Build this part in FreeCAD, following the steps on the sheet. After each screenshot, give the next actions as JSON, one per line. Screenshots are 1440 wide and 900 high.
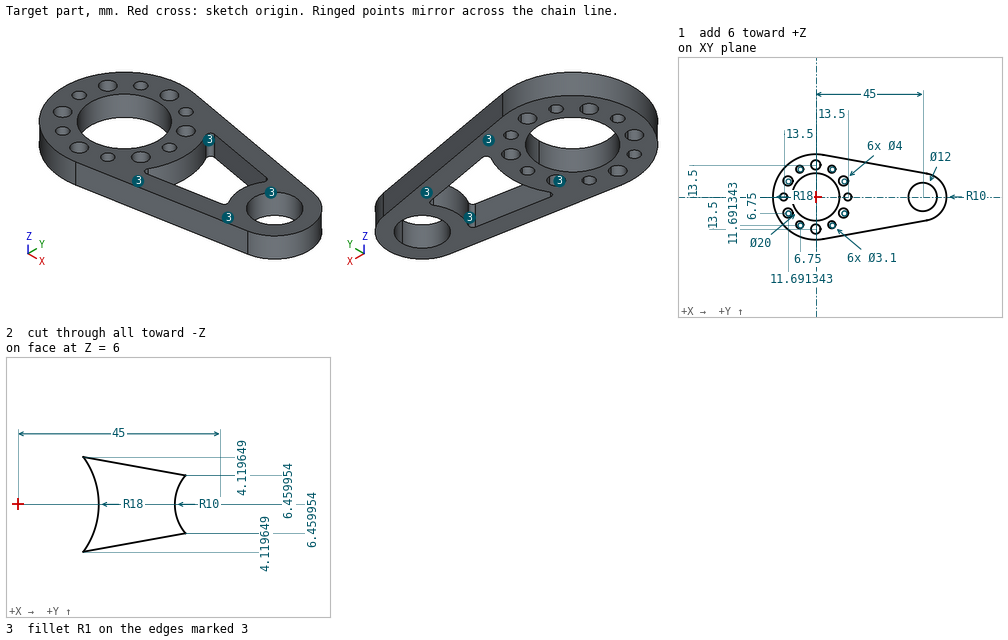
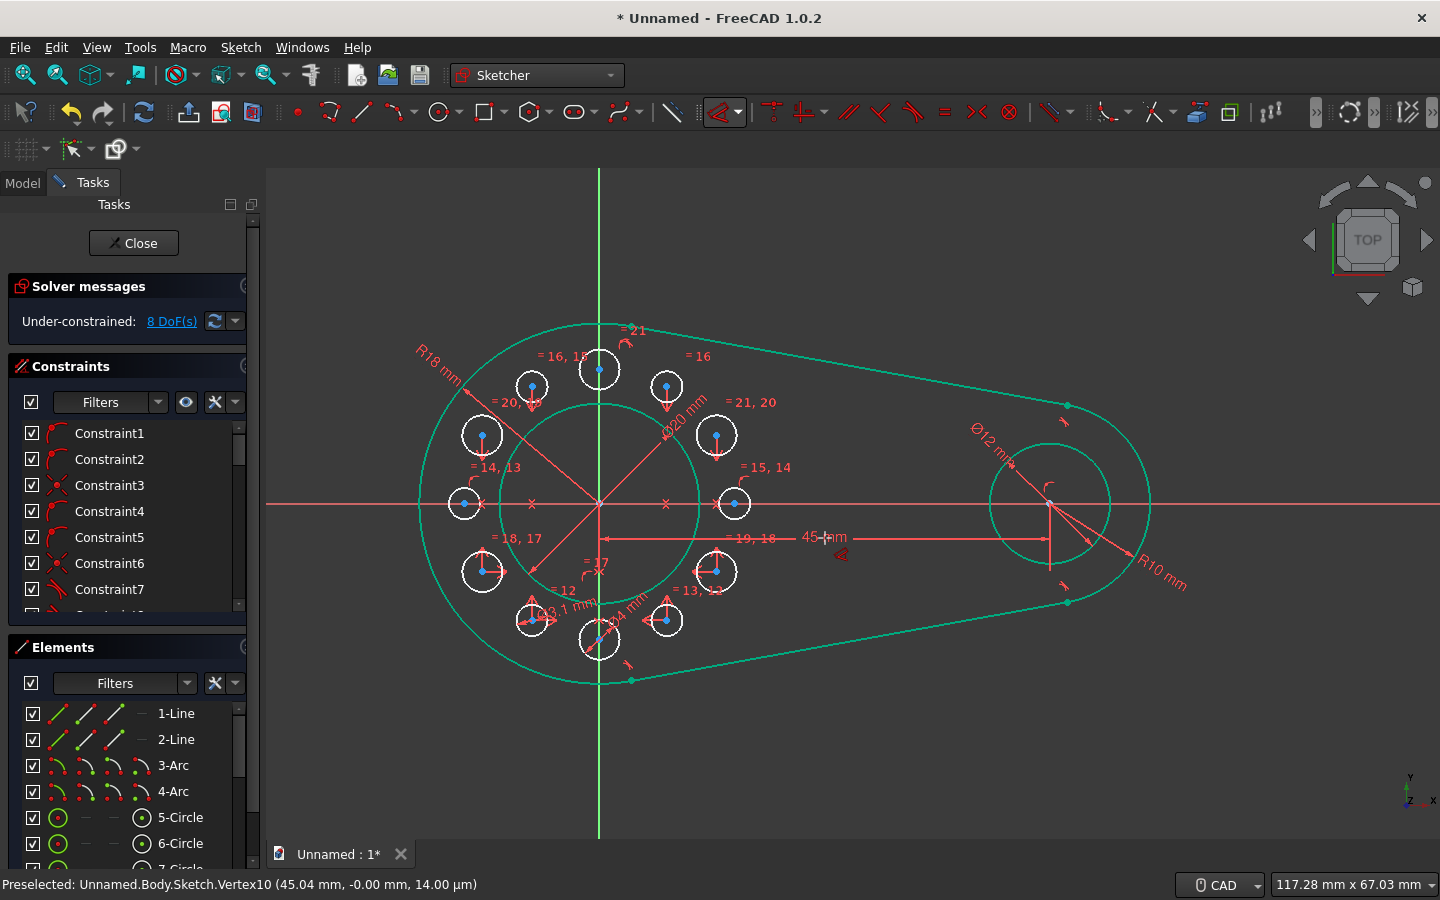
{"action": "left_click", "coordinate": [532, 620]}
{"action": "left_click", "coordinate": [566, 654]}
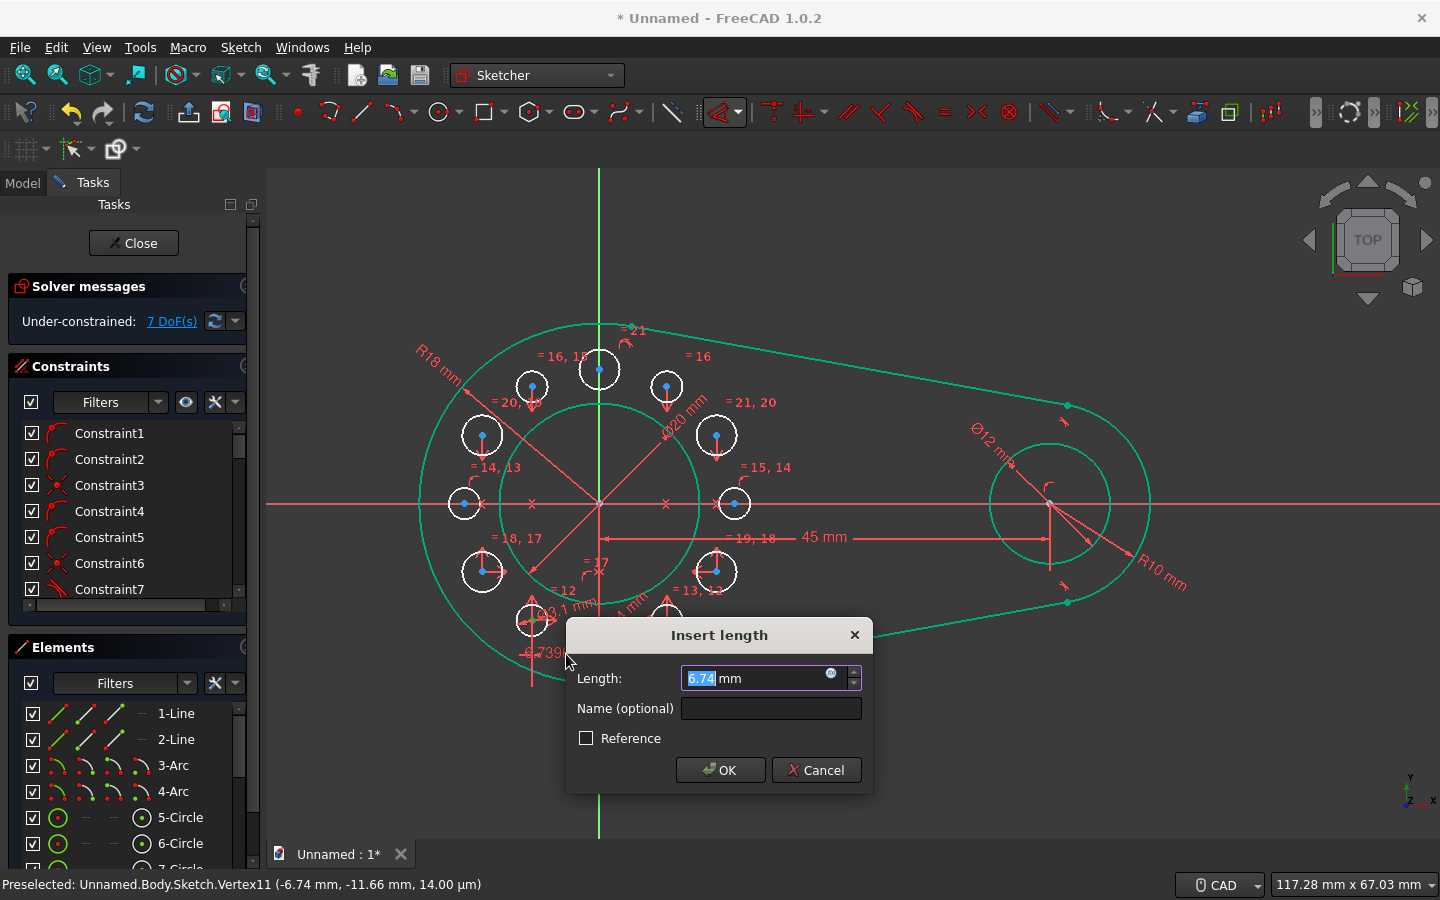
{"action": "type", "text": "6.75"}
{"action": "key", "text": "Return"}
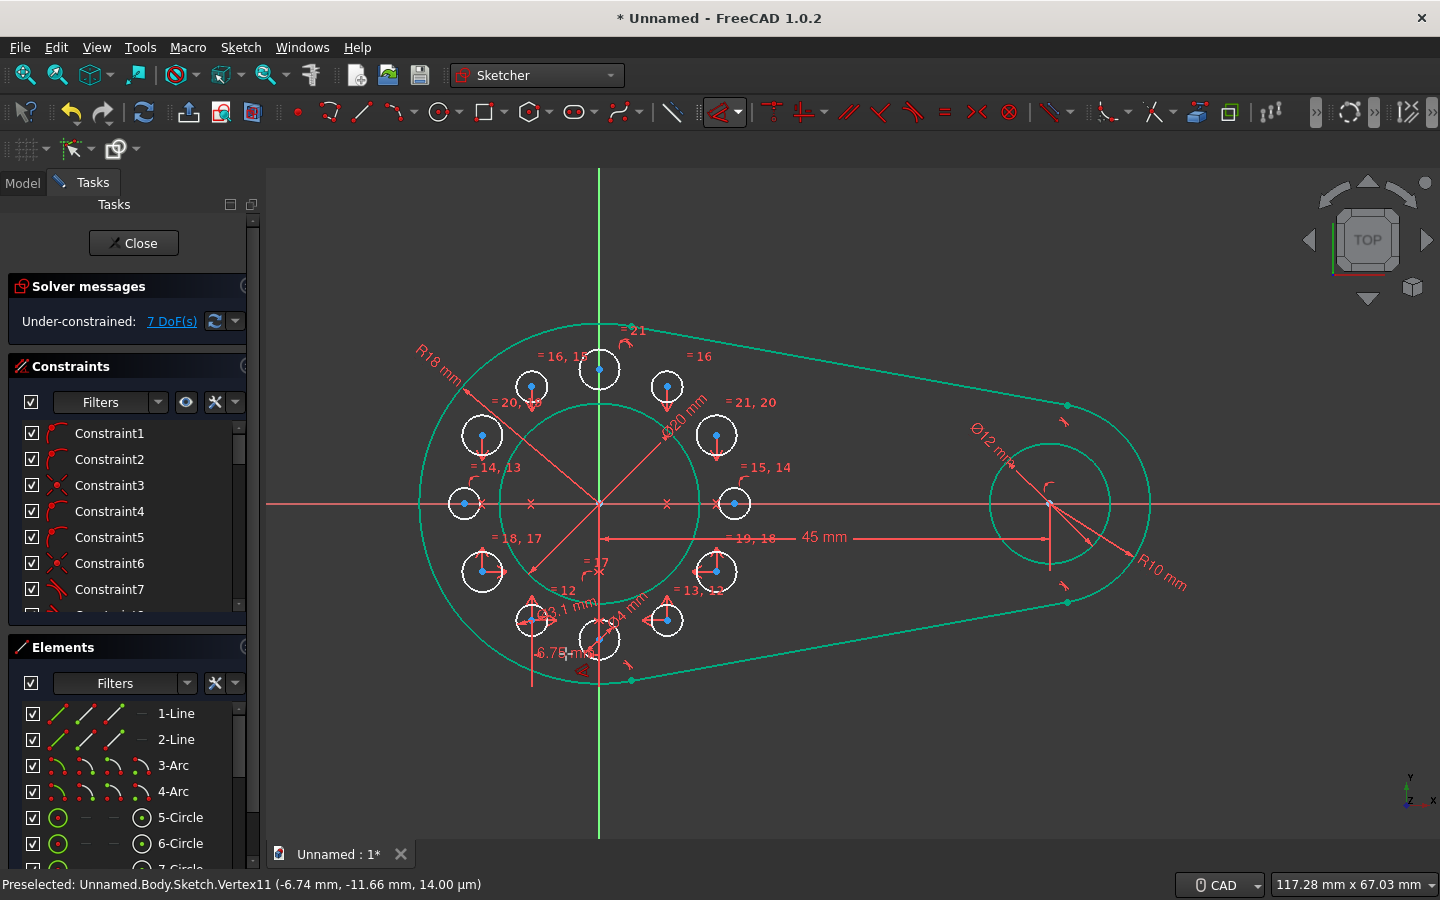
{"action": "left_click", "coordinate": [599, 640]}
{"action": "left_click", "coordinate": [565, 572]}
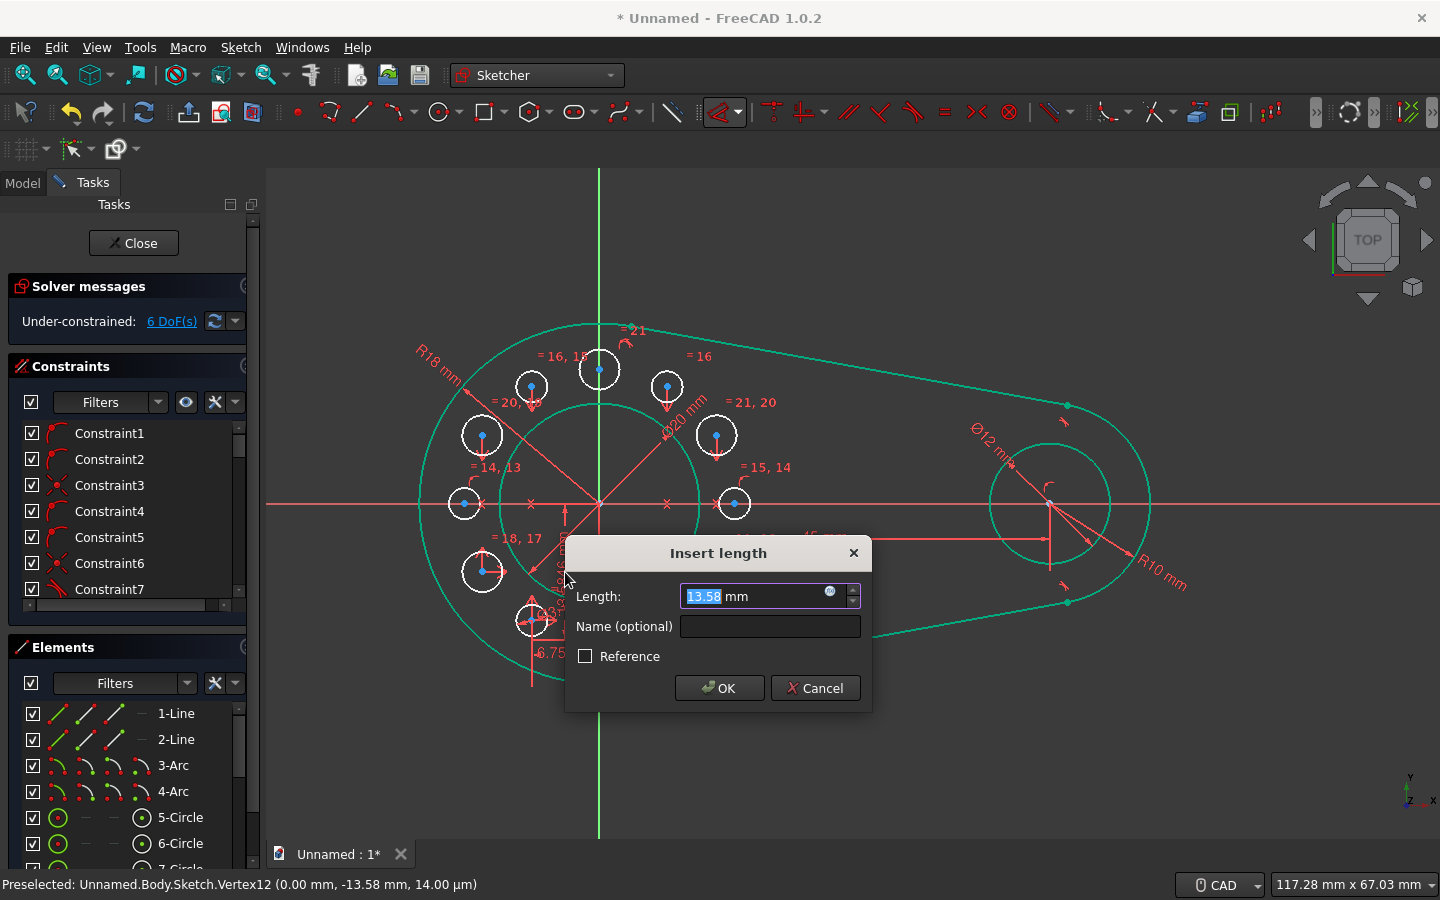
{"action": "type", "text": "13.5"}
{"action": "key", "text": "Return"}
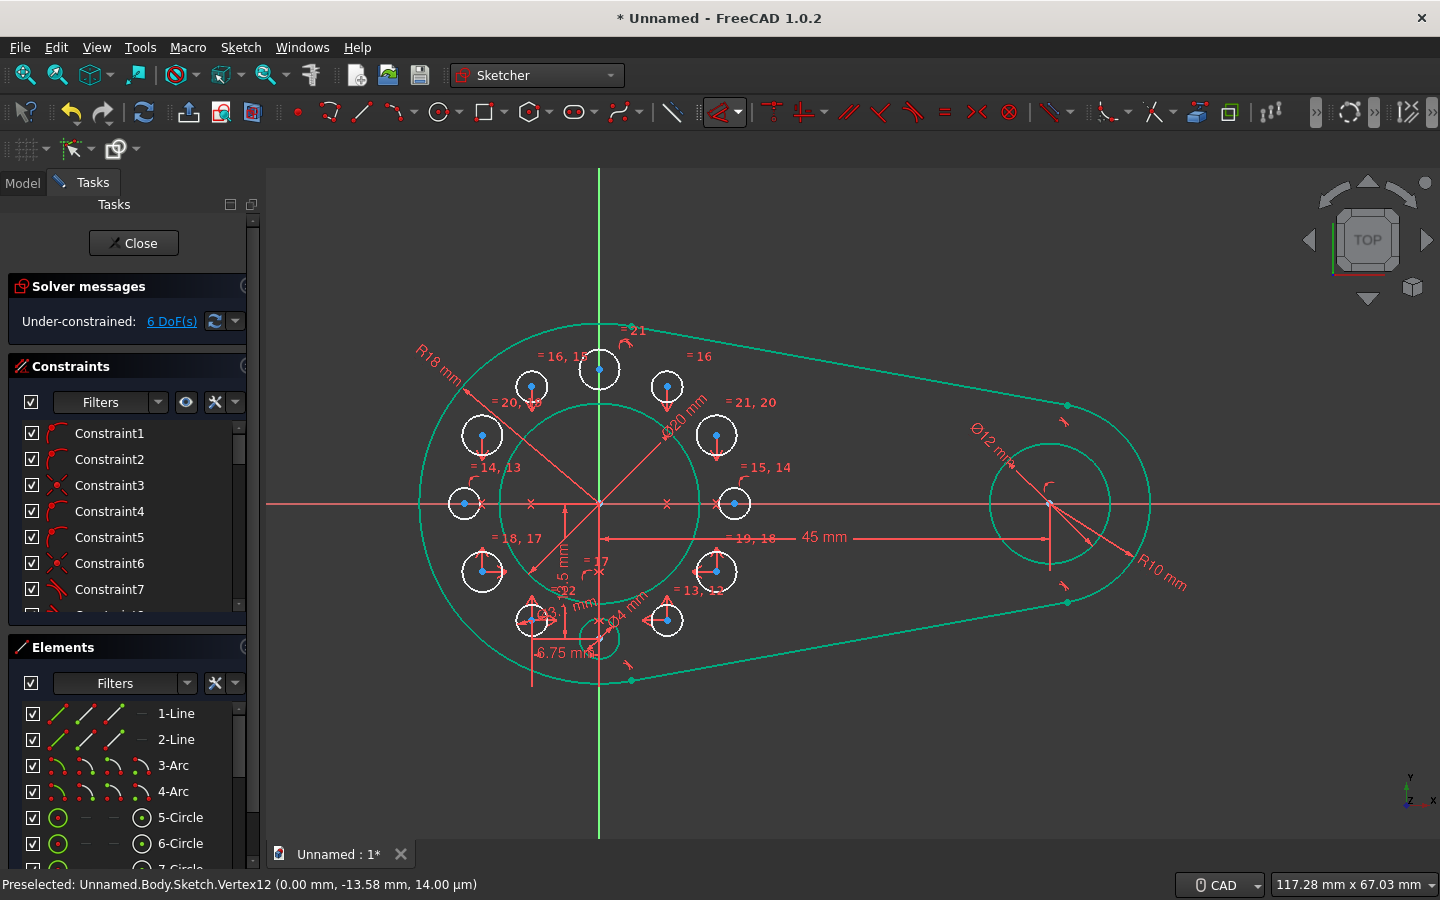
{"action": "left_click", "coordinate": [482, 572]}
{"action": "left_click", "coordinate": [448, 538]}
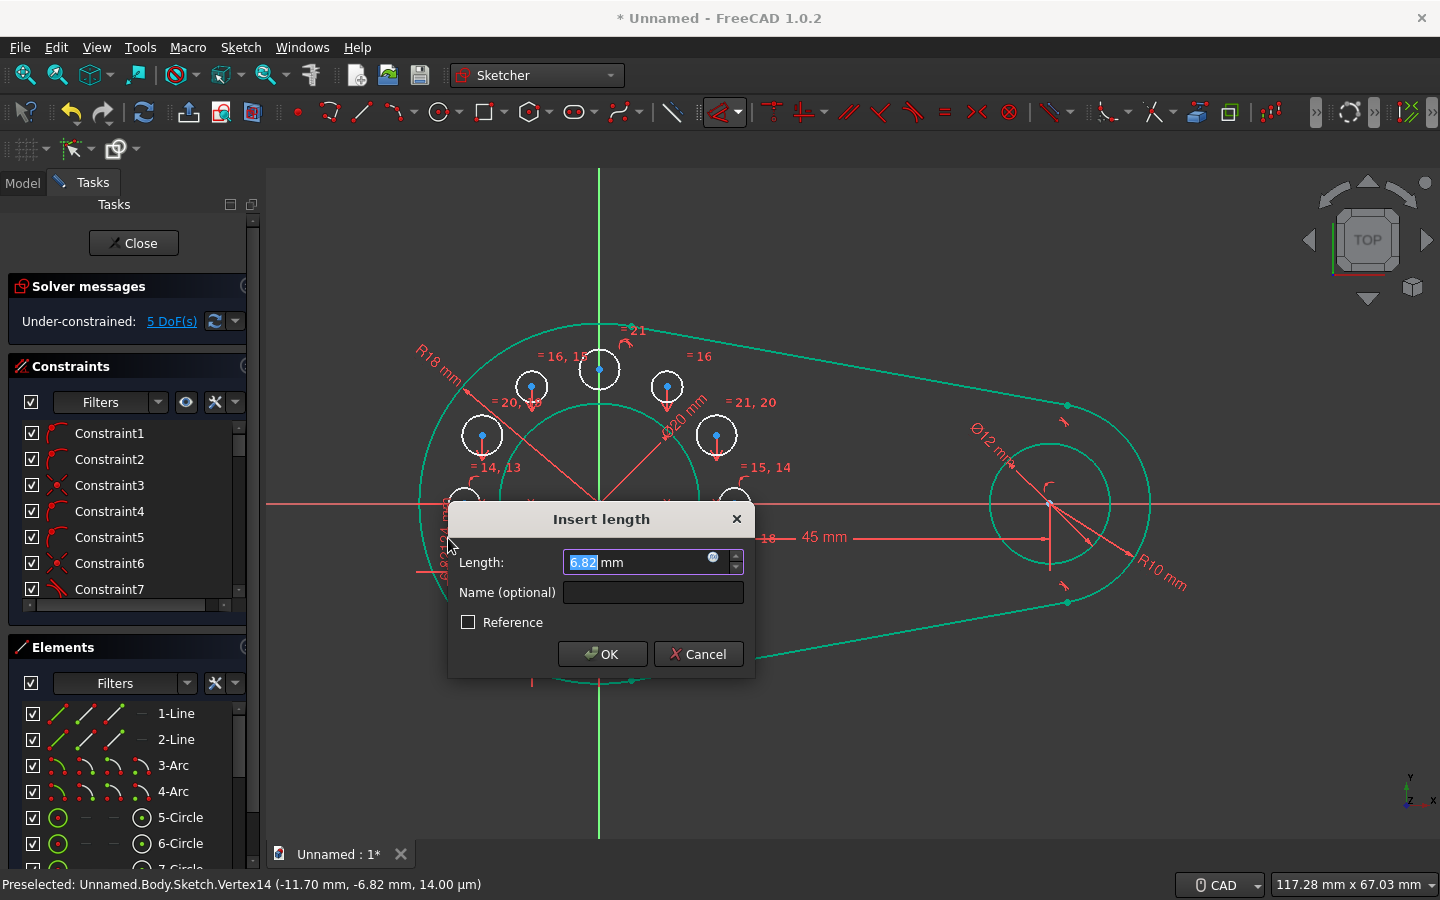
{"action": "type", "text": "6.75"}
{"action": "key", "text": "Return"}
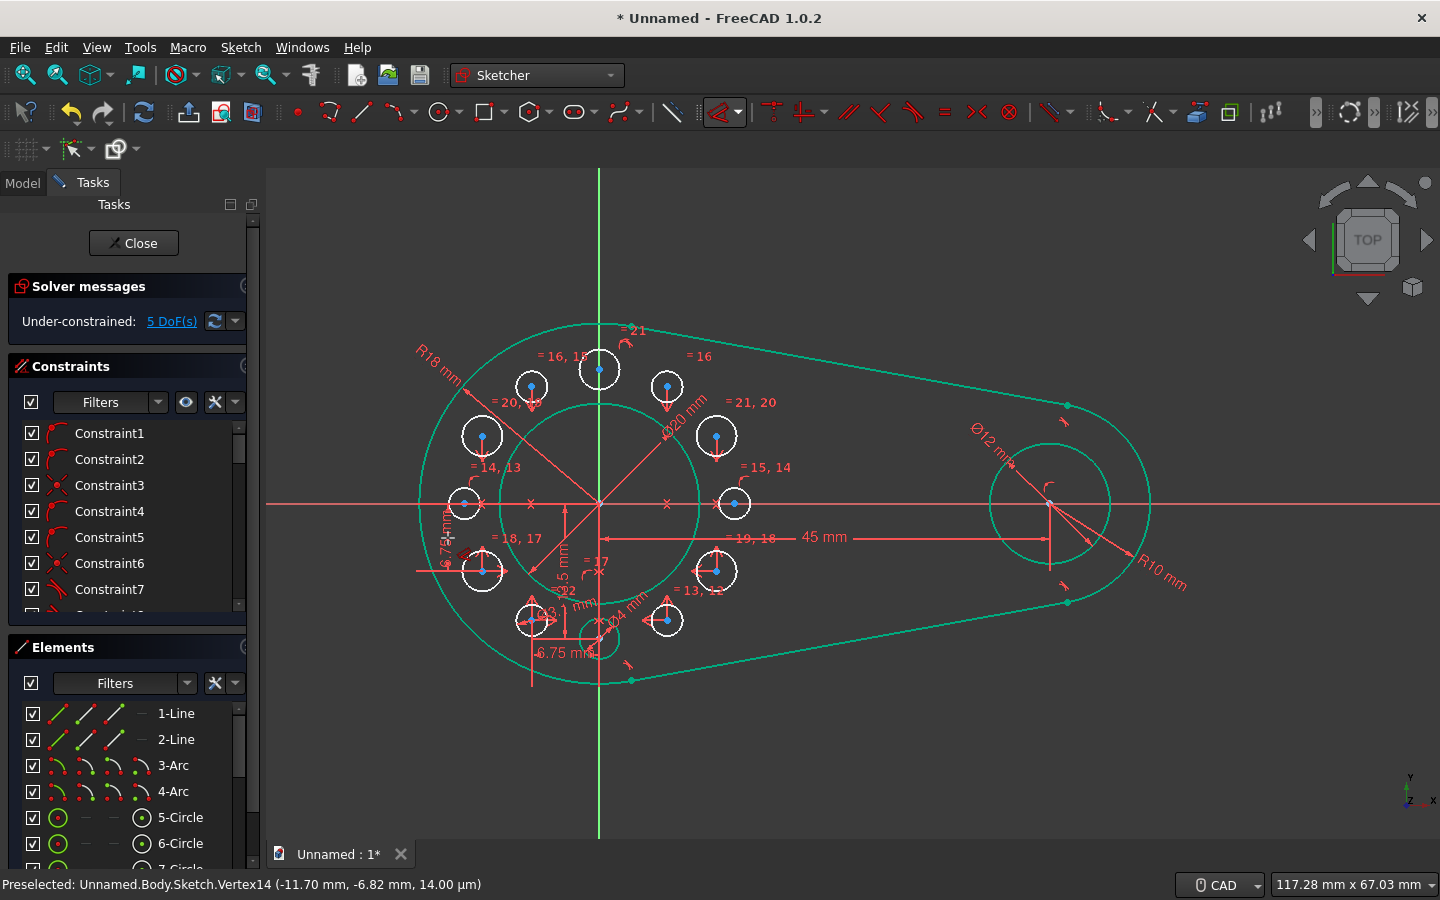
{"action": "left_click", "coordinate": [465, 504]}
{"action": "left_click", "coordinate": [532, 538]}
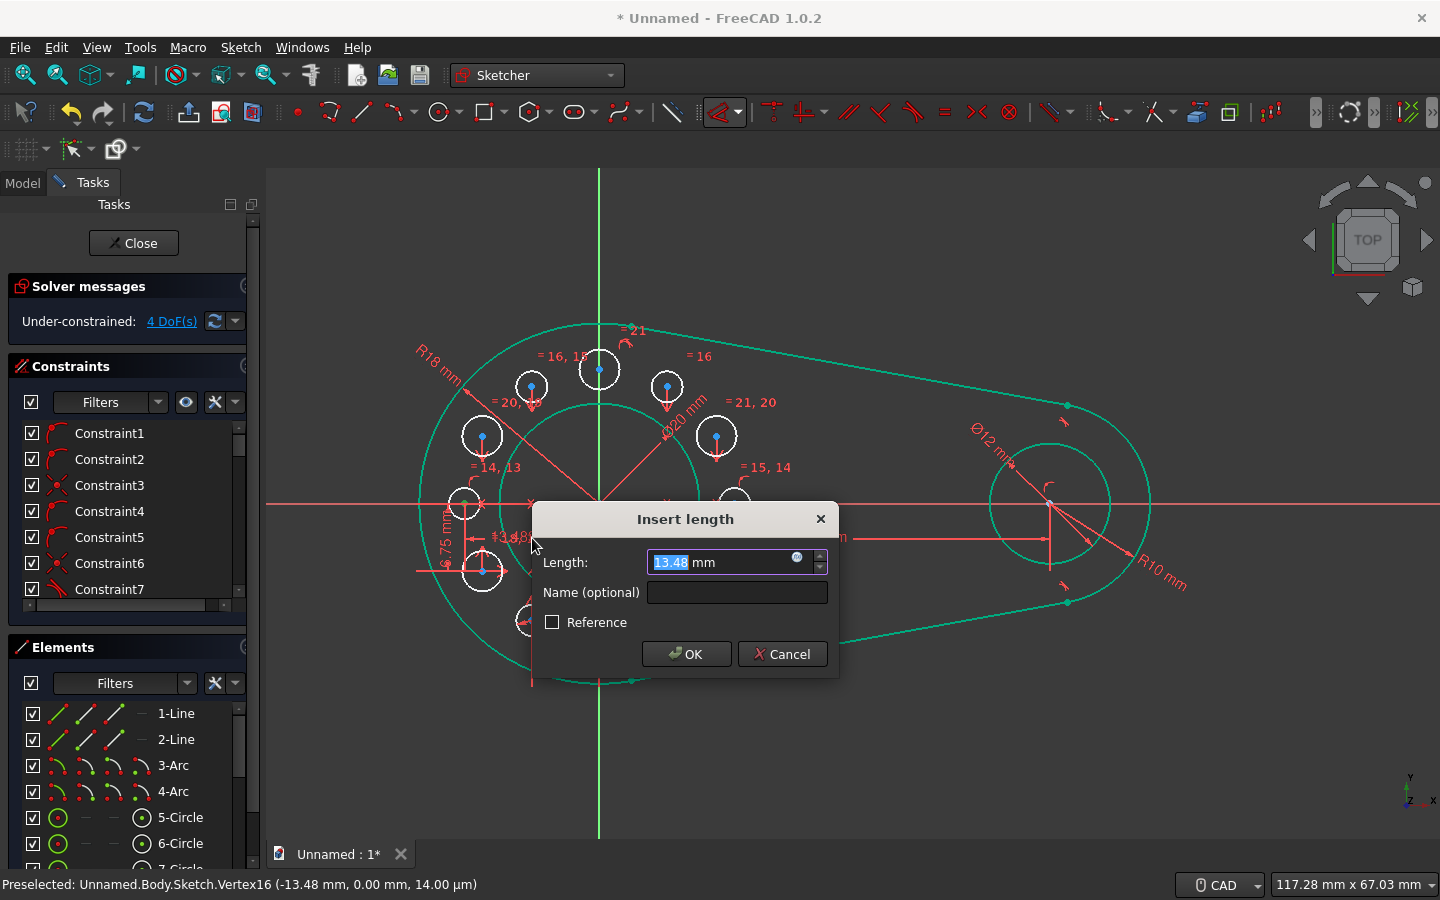
{"action": "type", "text": "13.5"}
{"action": "key", "text": "Return"}